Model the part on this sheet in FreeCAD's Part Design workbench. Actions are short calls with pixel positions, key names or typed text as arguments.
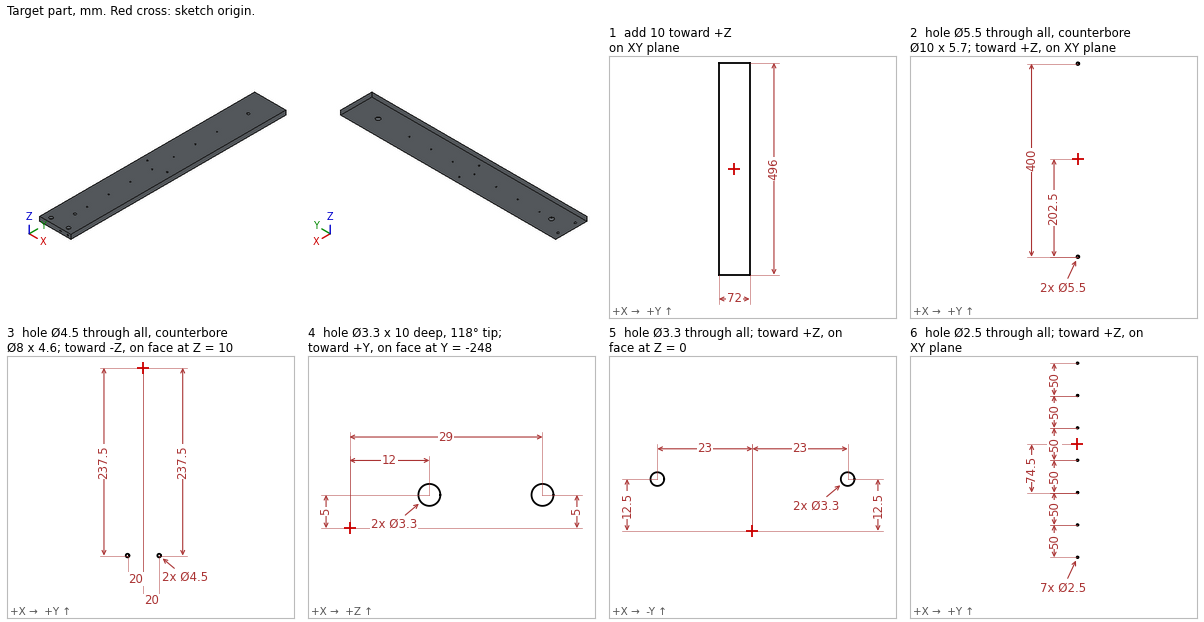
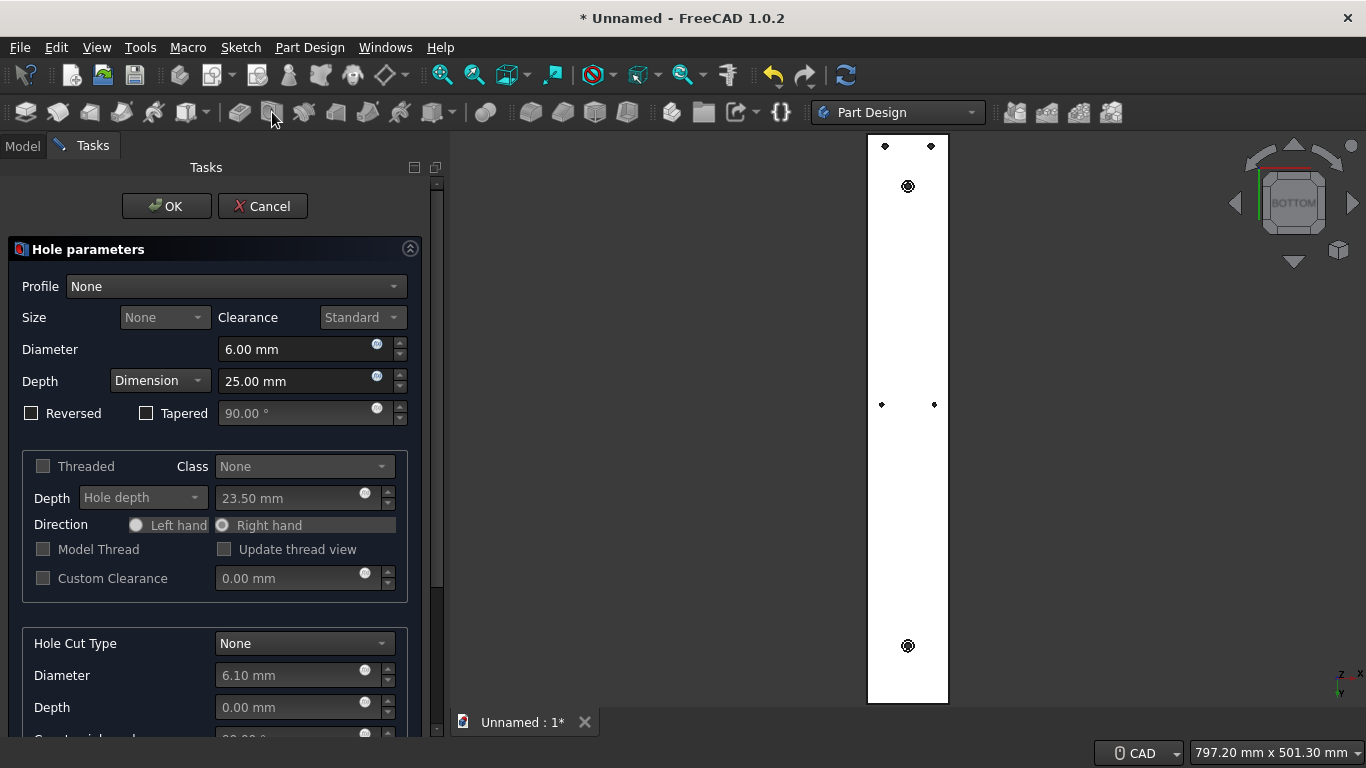
triple_click(305, 349)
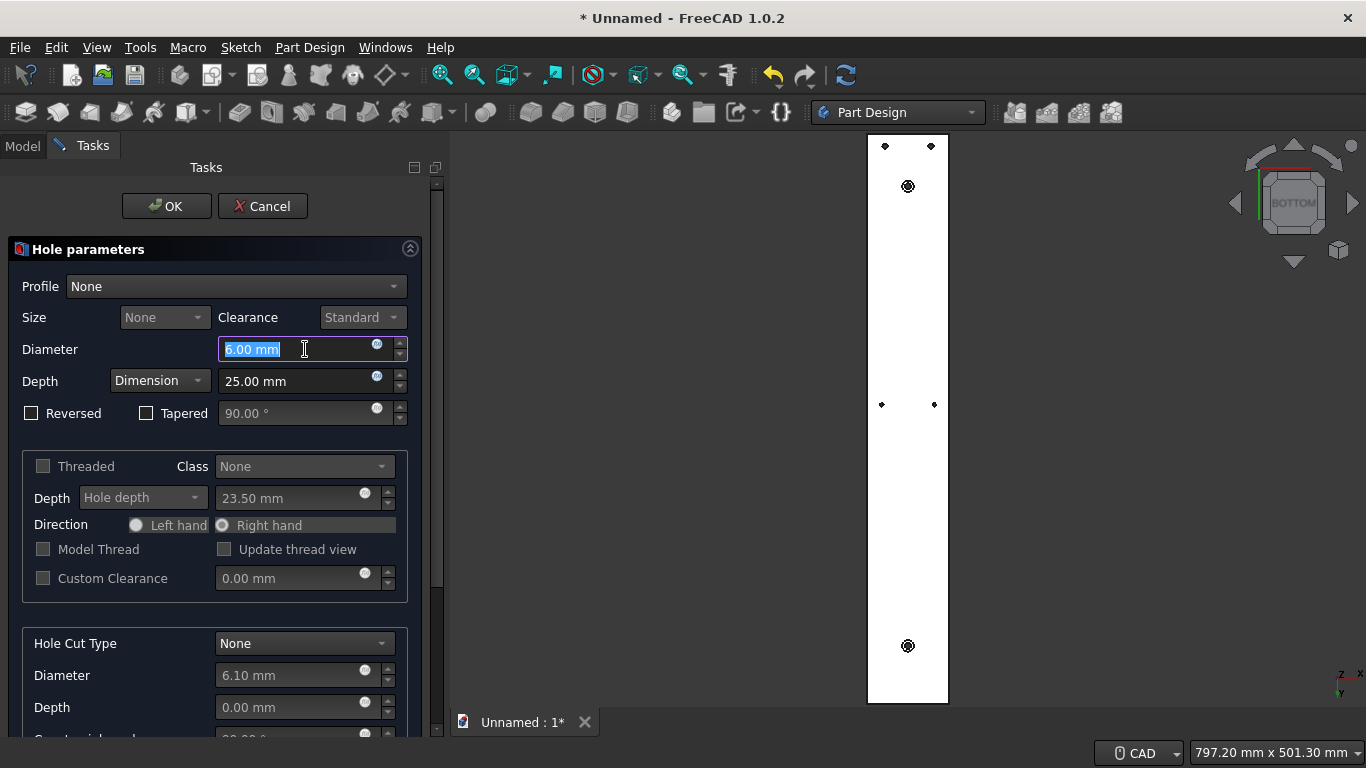
text(2.5)
key(Tab)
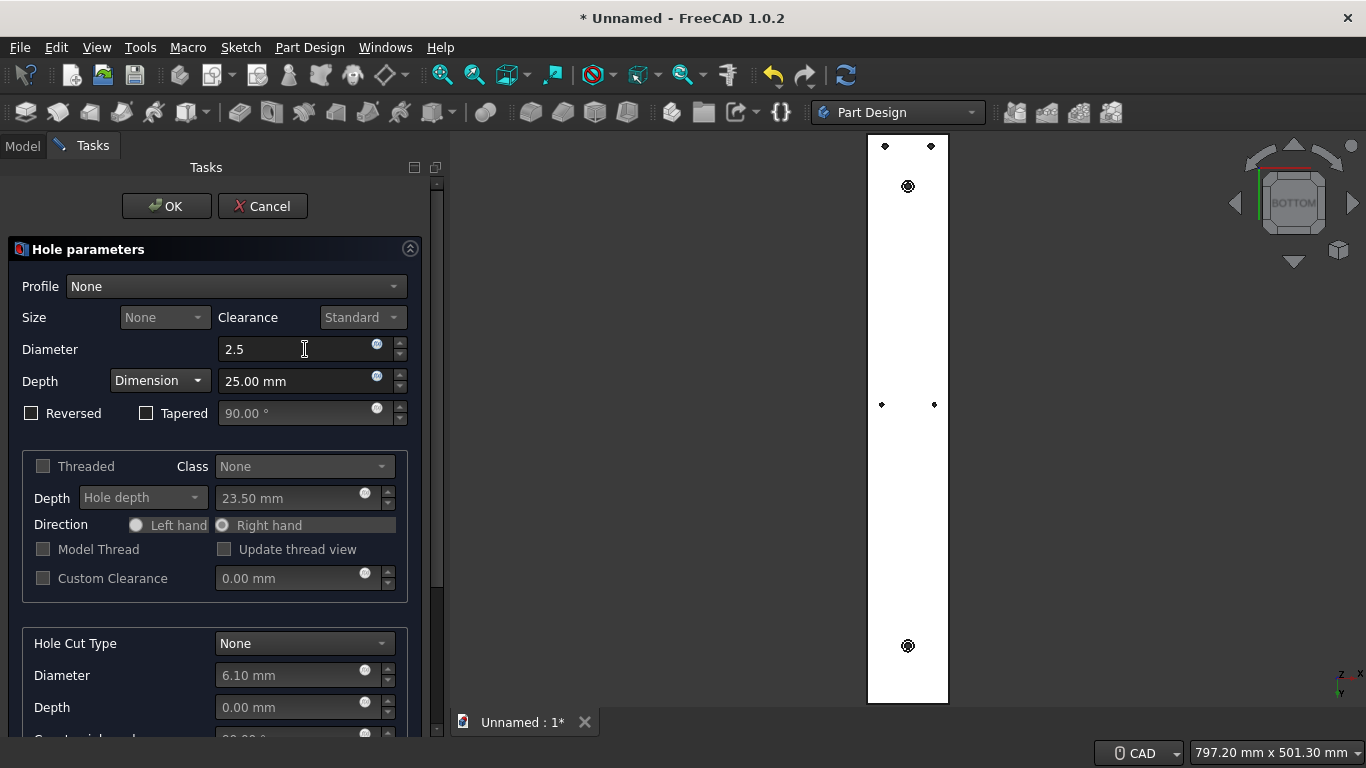
click(161, 380)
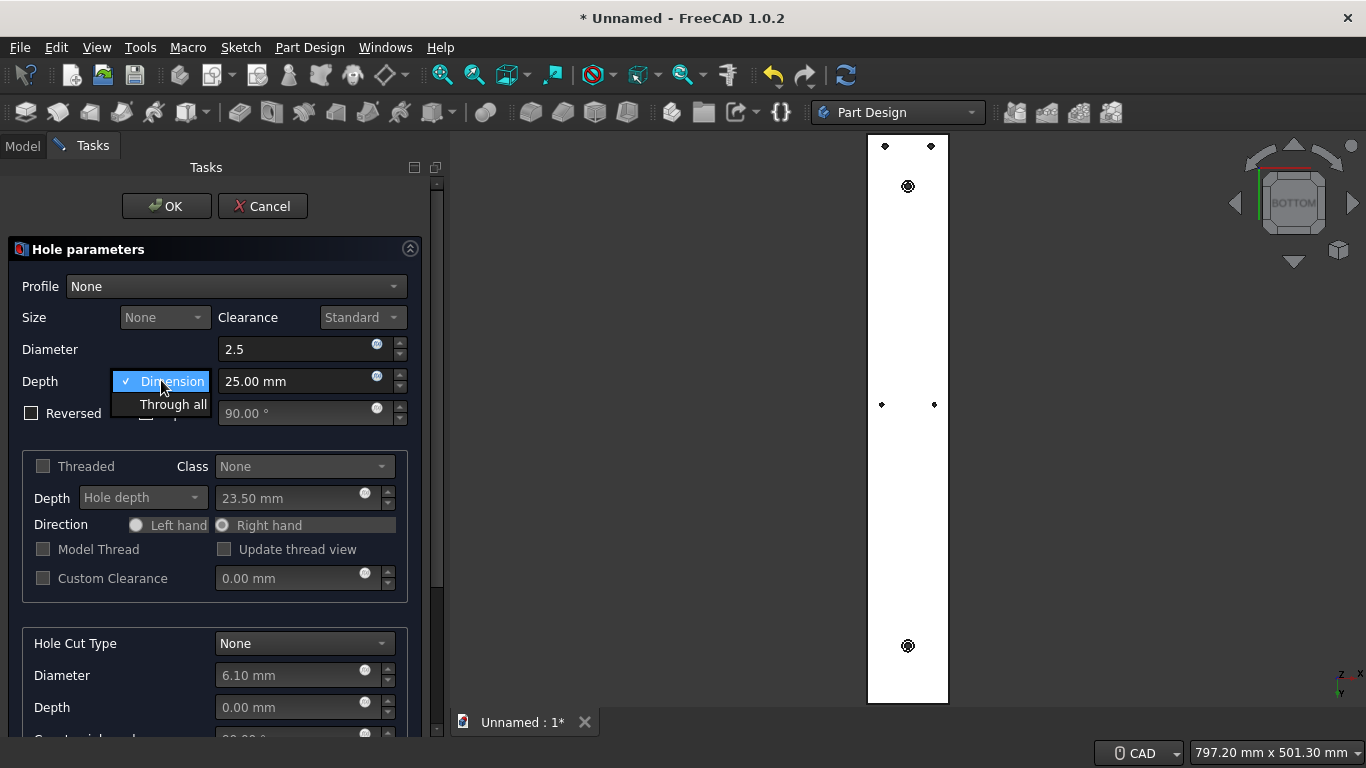
click(160, 404)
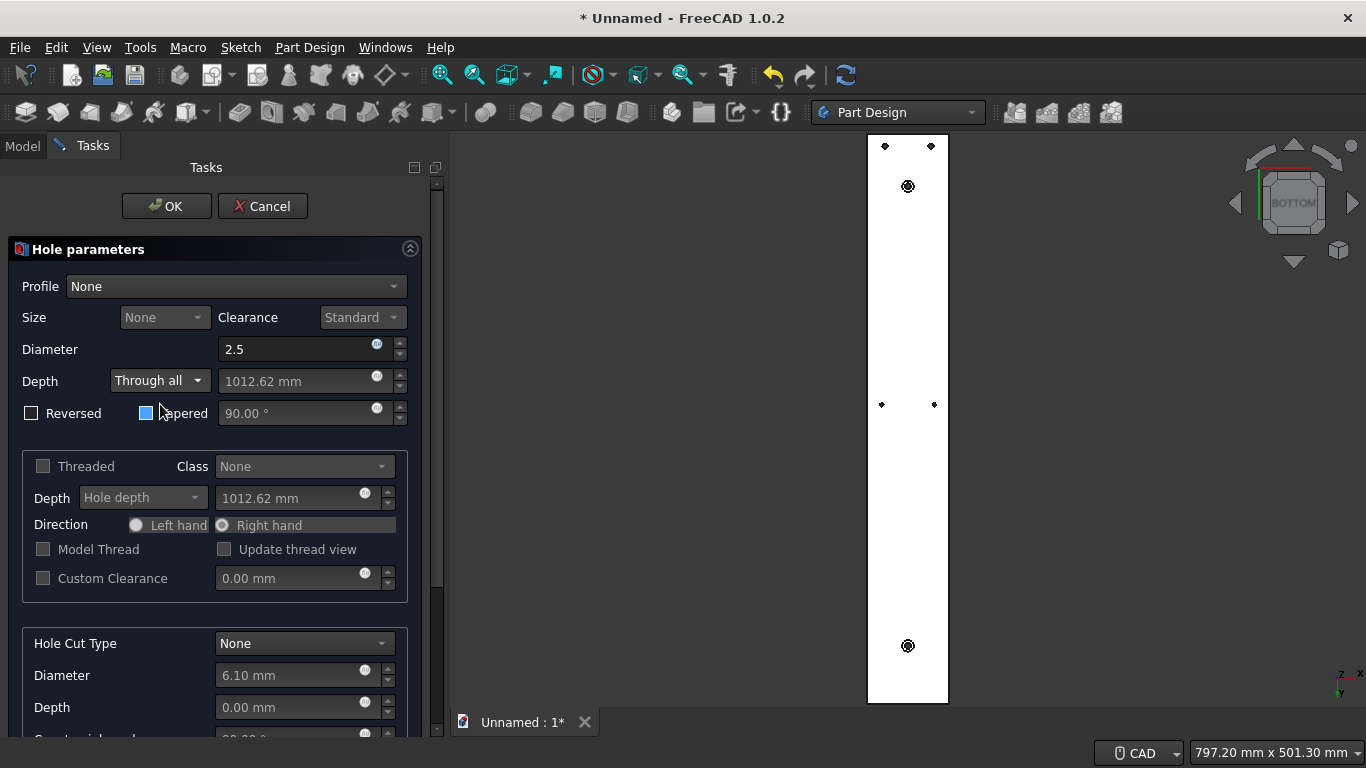
click(30, 413)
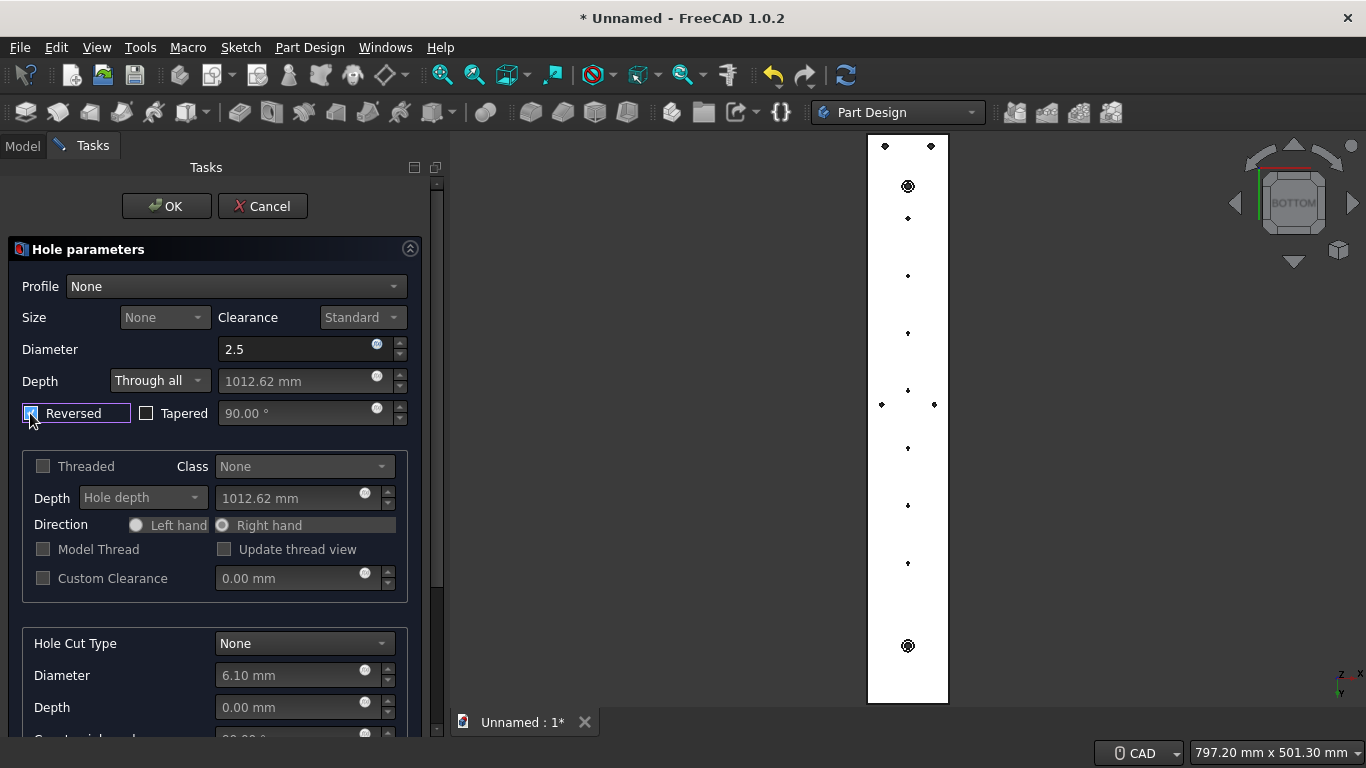
click(167, 206)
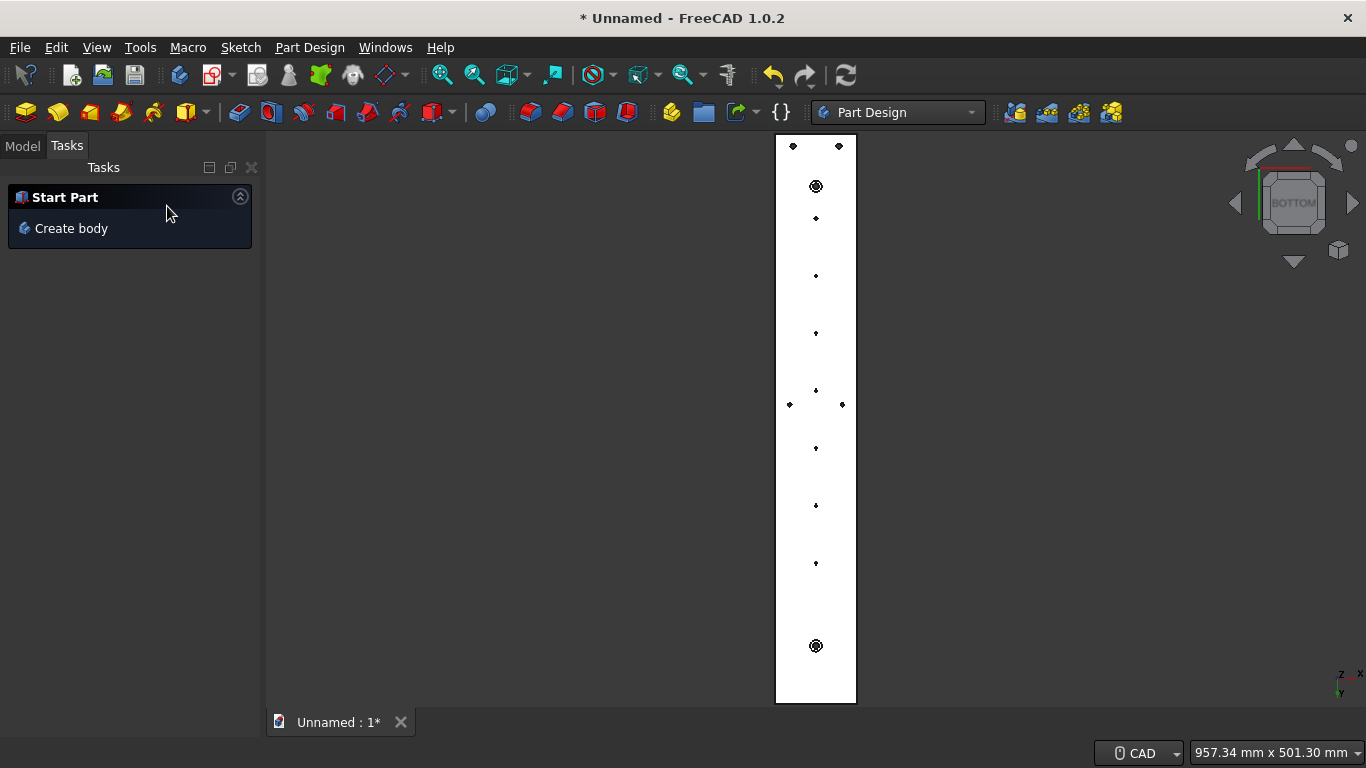
key(0)